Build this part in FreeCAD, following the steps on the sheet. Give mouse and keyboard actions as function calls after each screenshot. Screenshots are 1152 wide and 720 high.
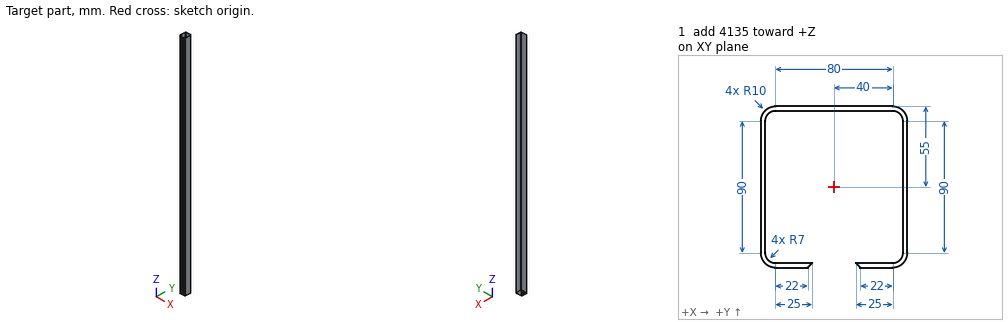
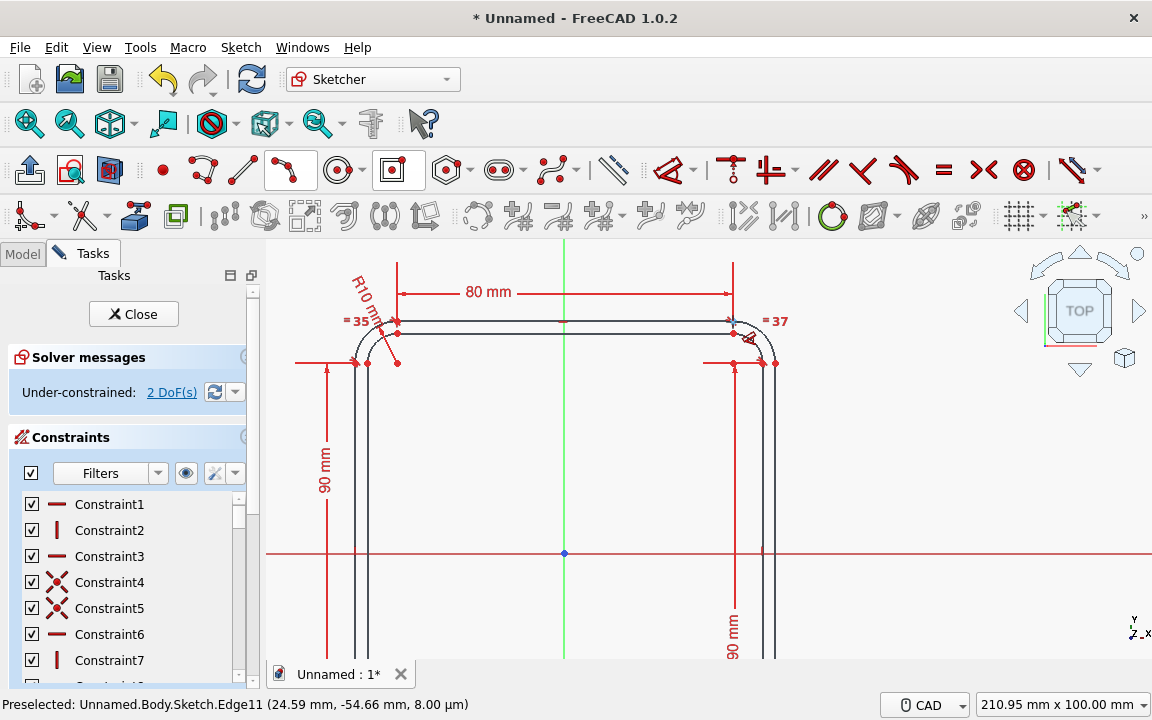
click(733, 321)
click(649, 287)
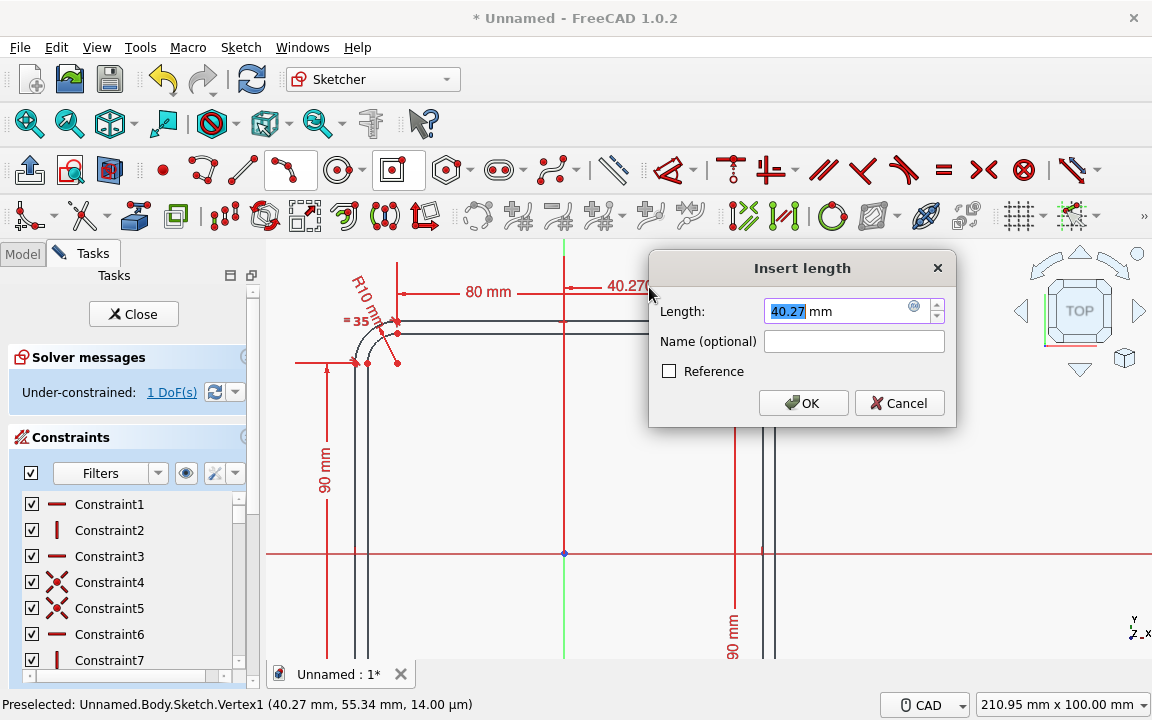
text(40)
key(Return)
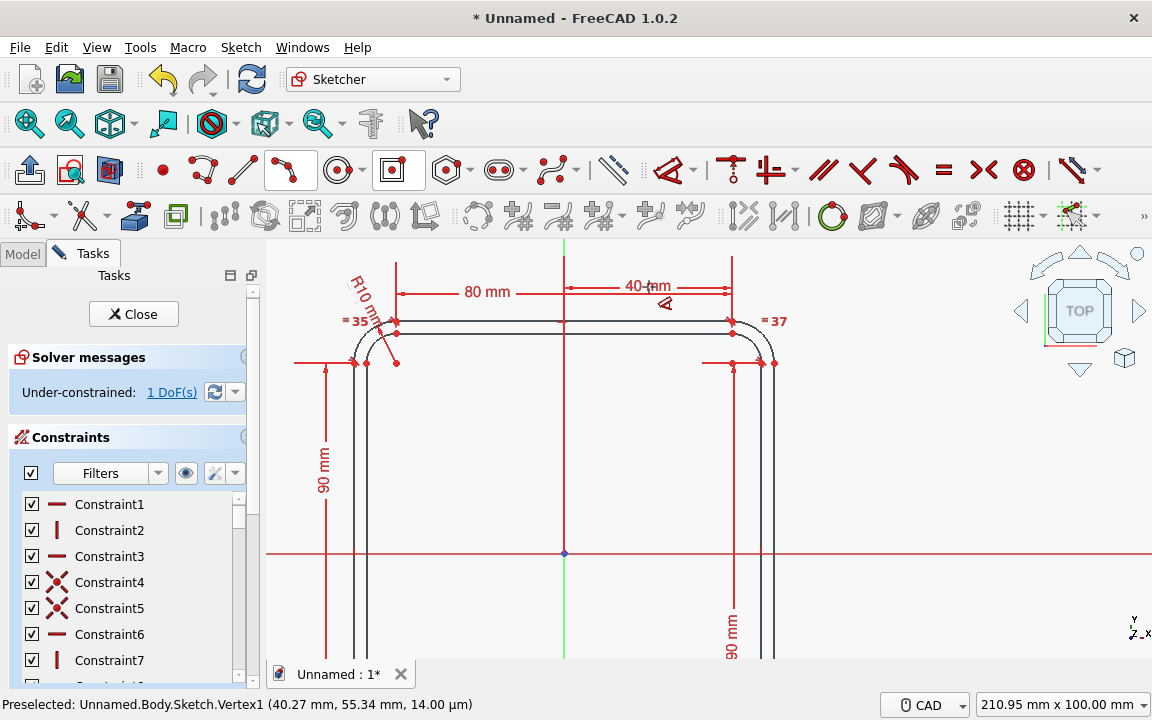
click(732, 321)
click(530, 438)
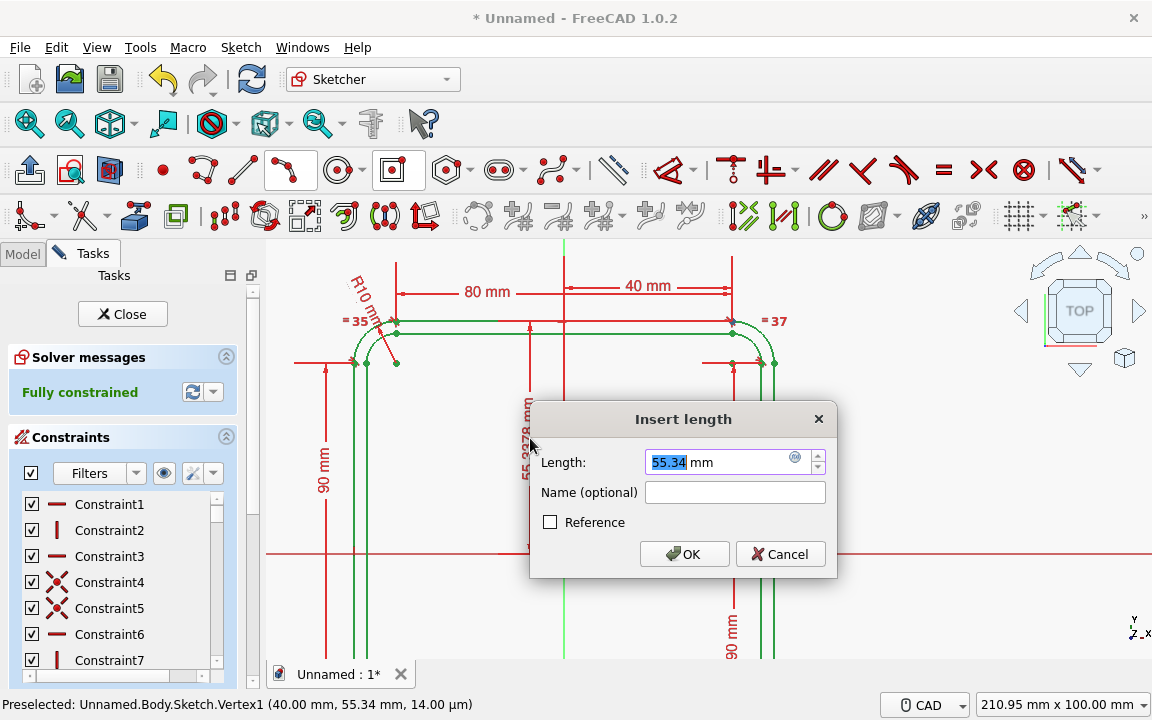
text(55)
key(Return)
key(Escape)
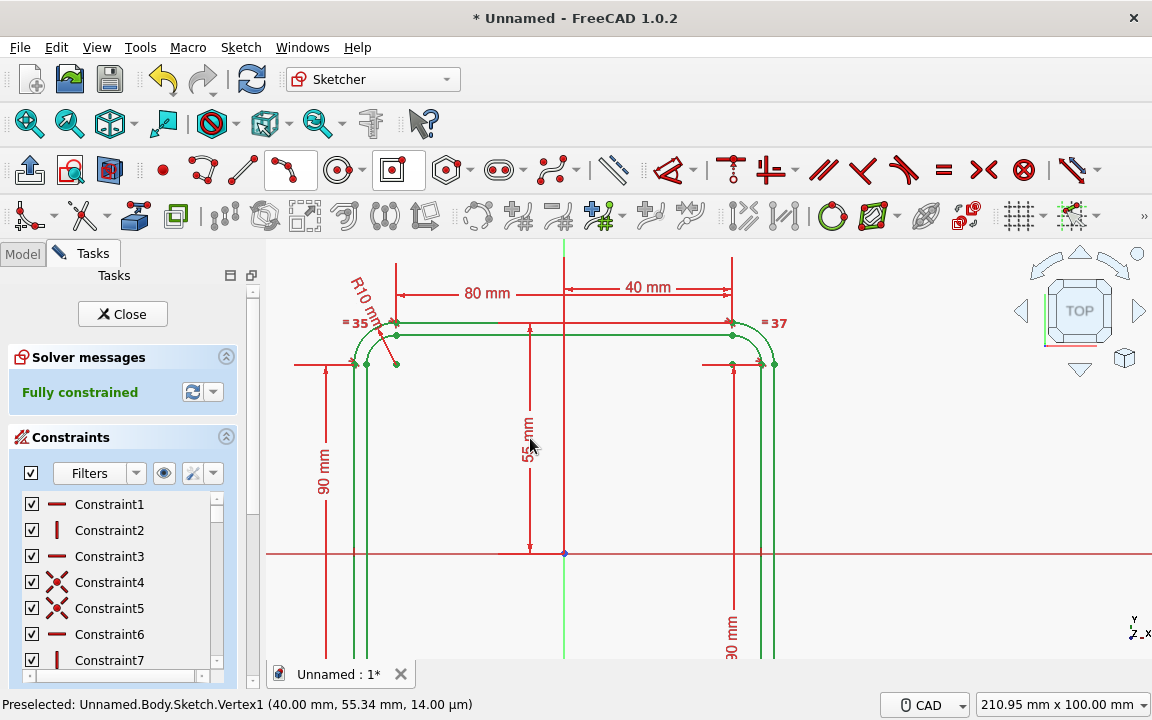
click(123, 314)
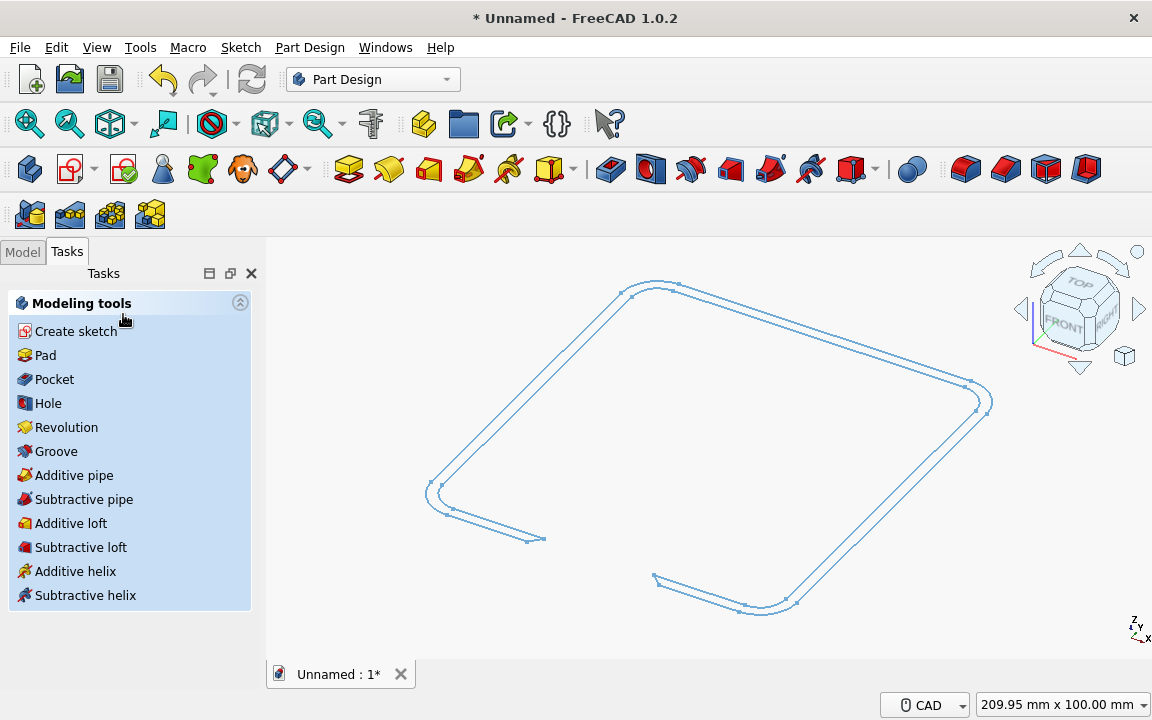
click(350, 170)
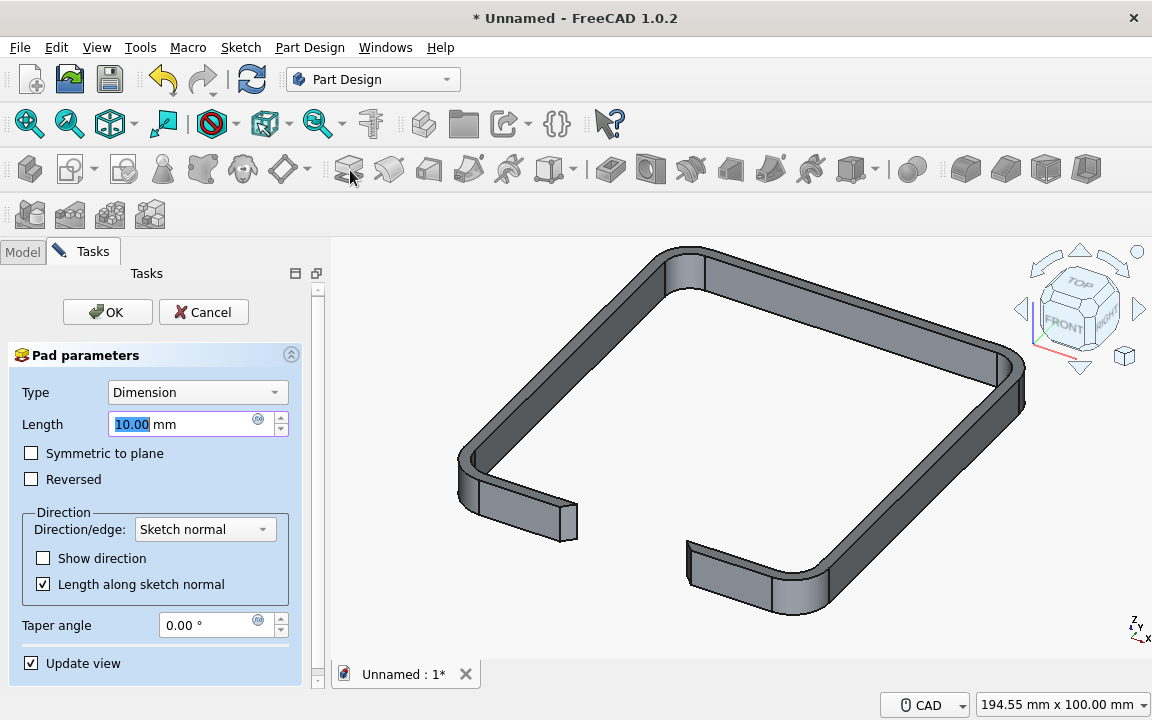
text(4135)
key(Tab)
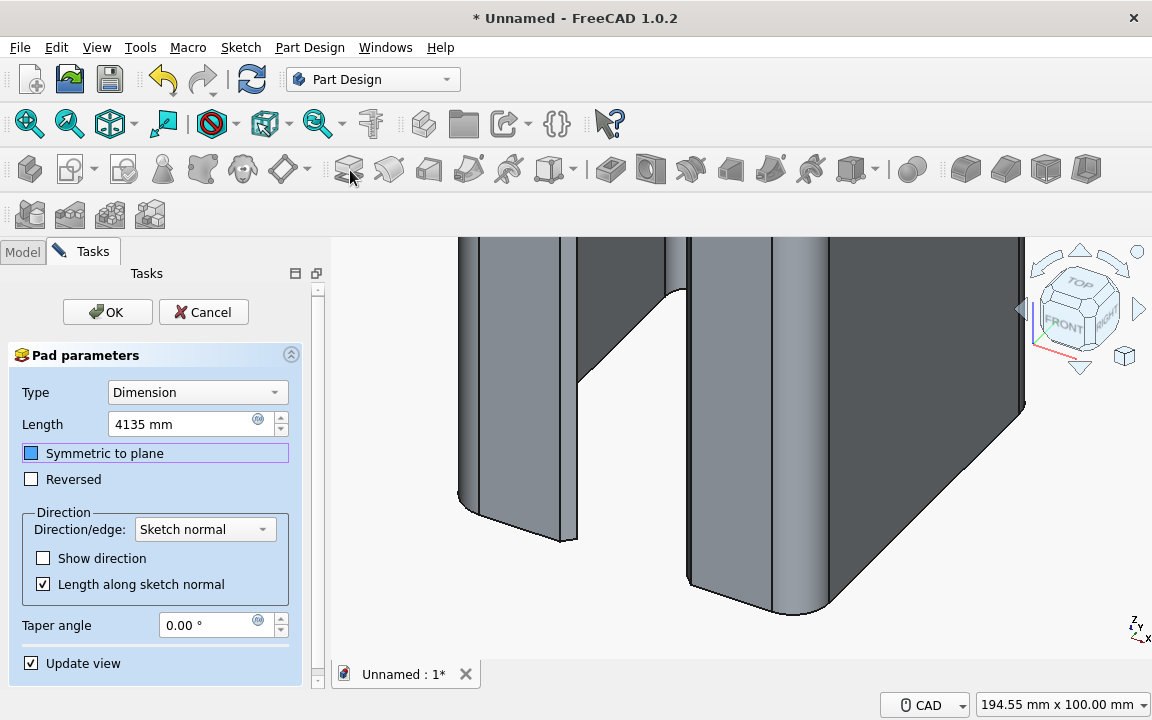
click(108, 312)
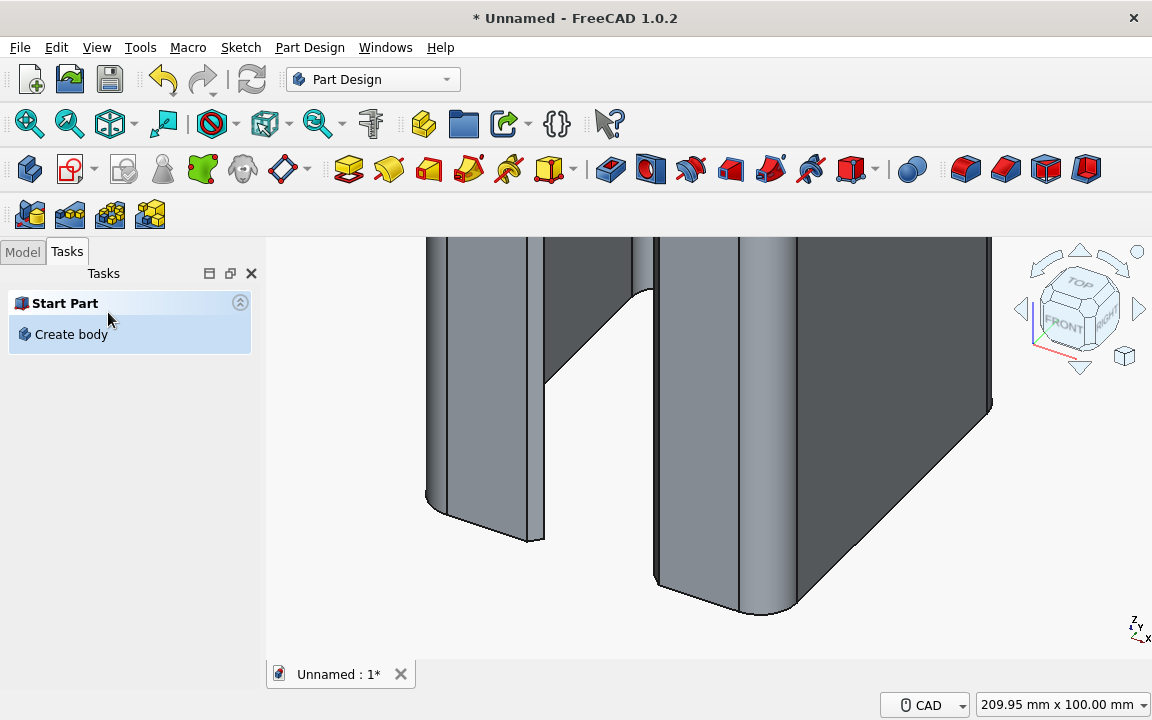
key(0)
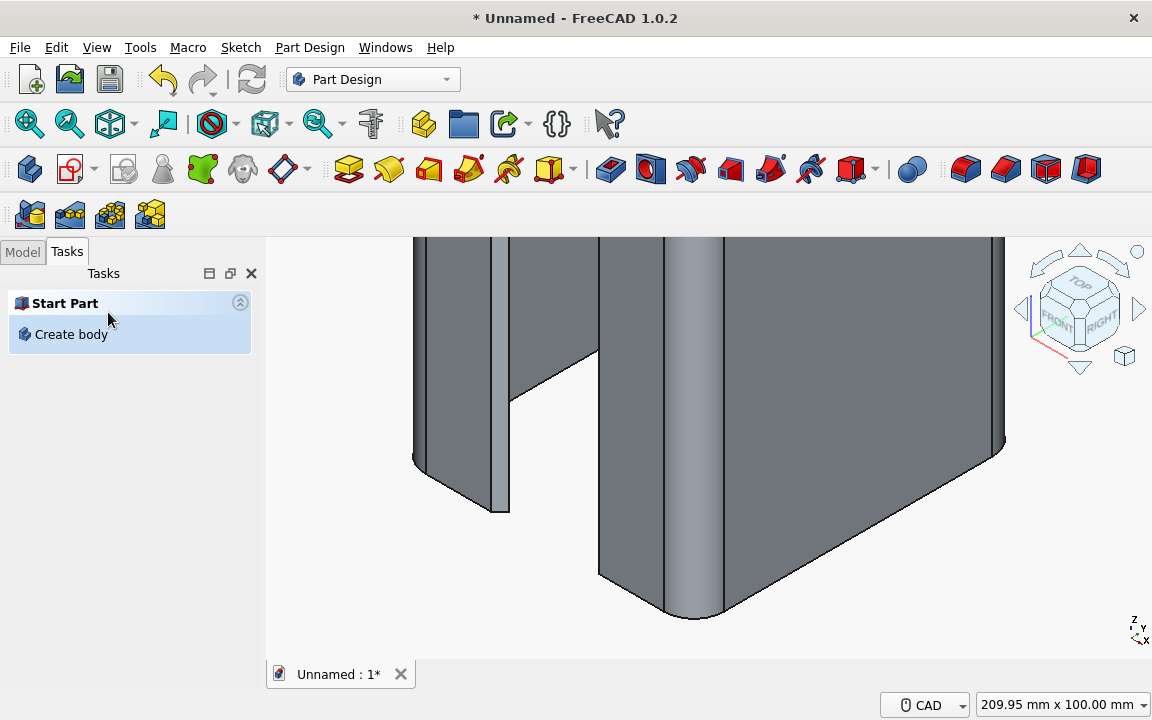
click(30, 124)